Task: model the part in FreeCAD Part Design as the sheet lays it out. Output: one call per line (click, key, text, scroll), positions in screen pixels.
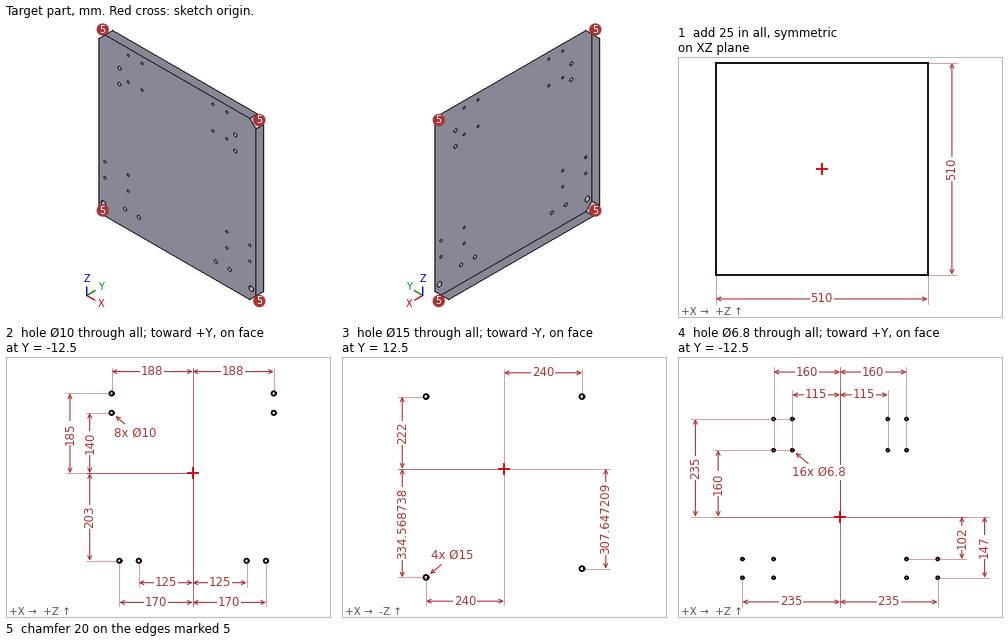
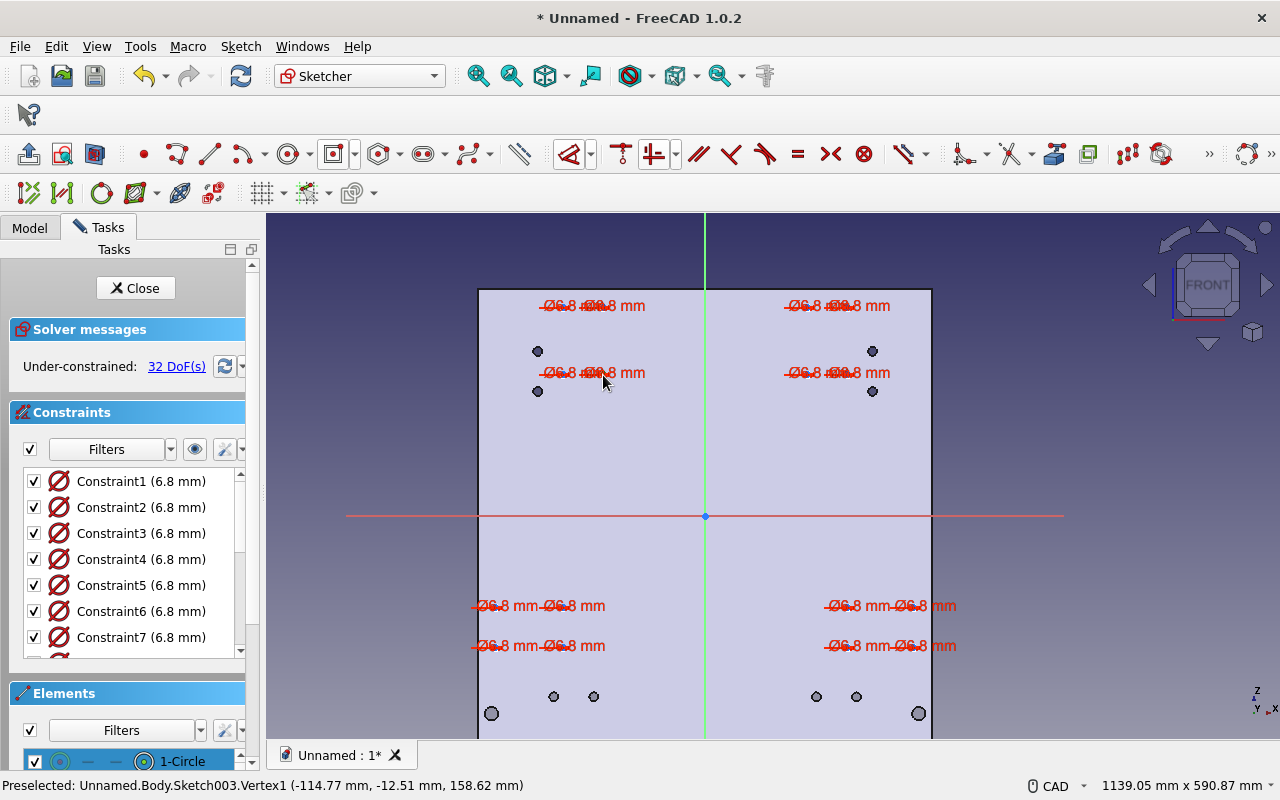
click(563, 375)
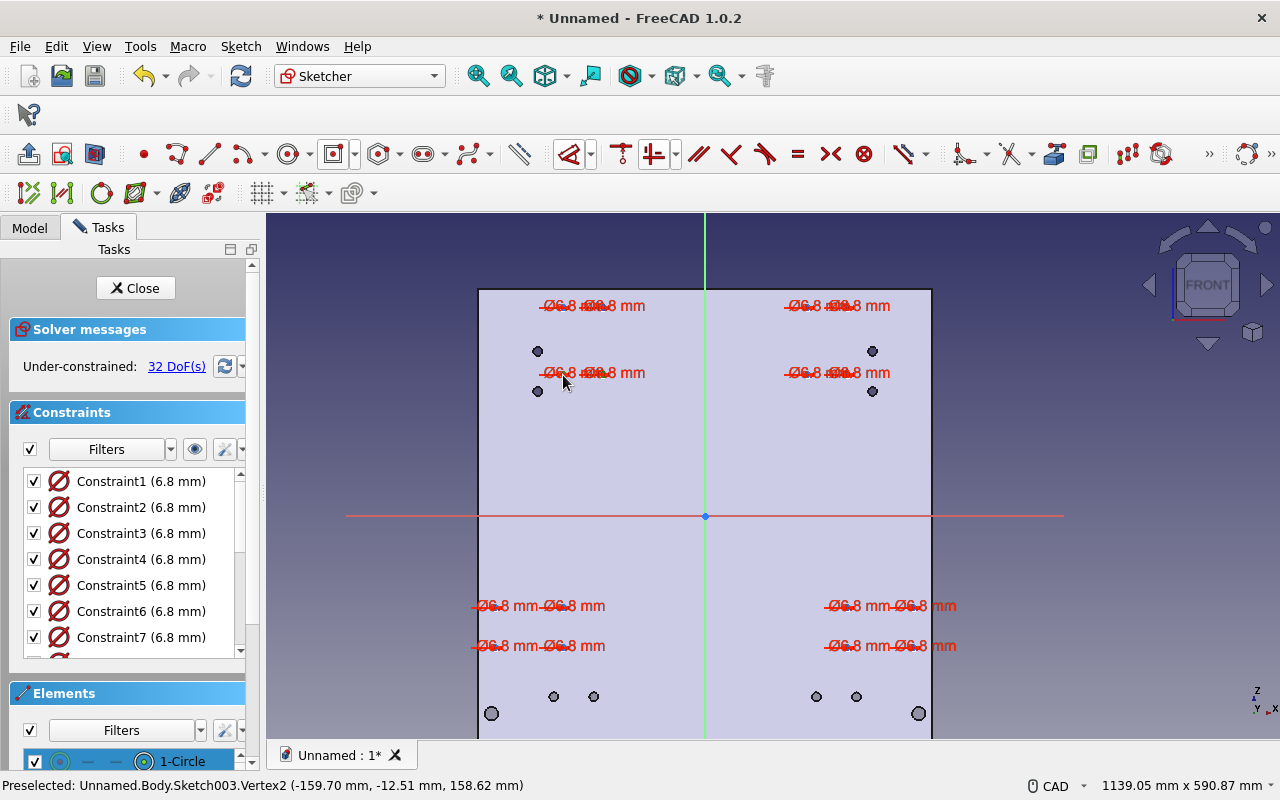
click(676, 154)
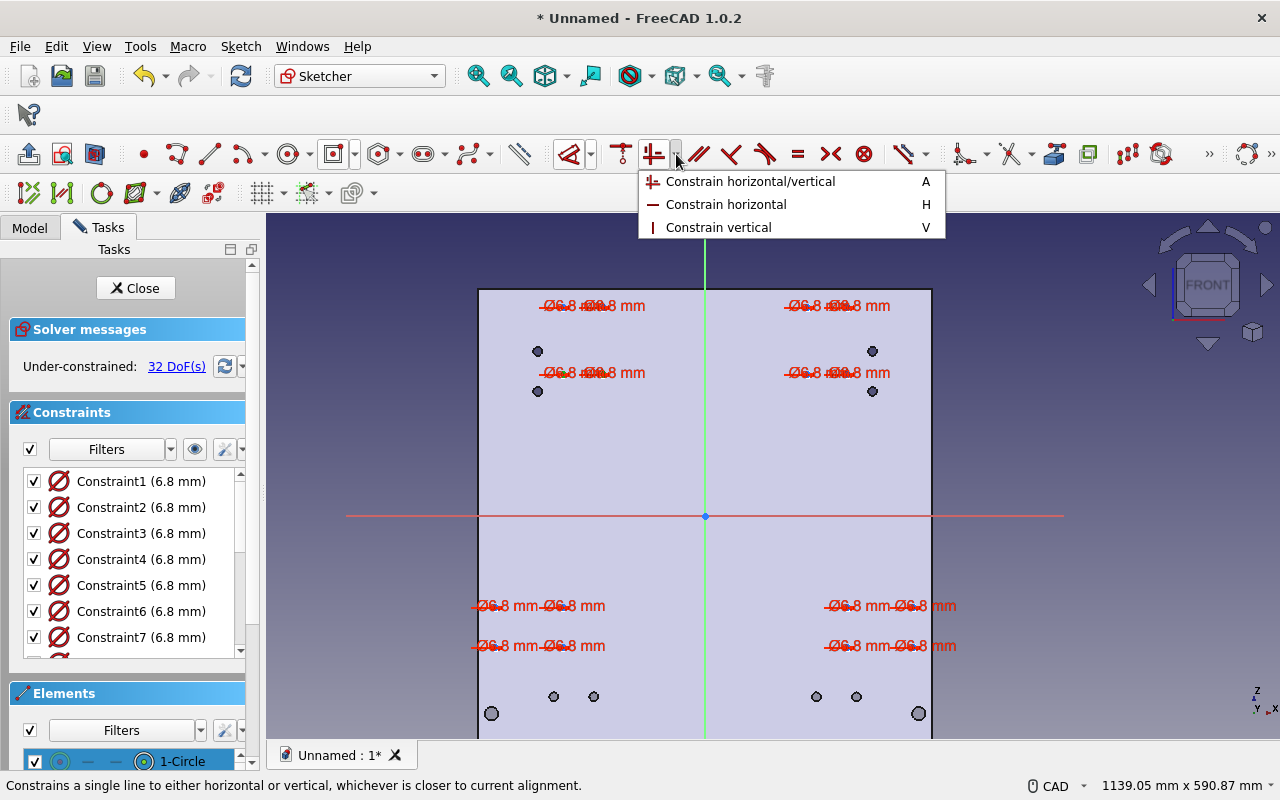
click(792, 204)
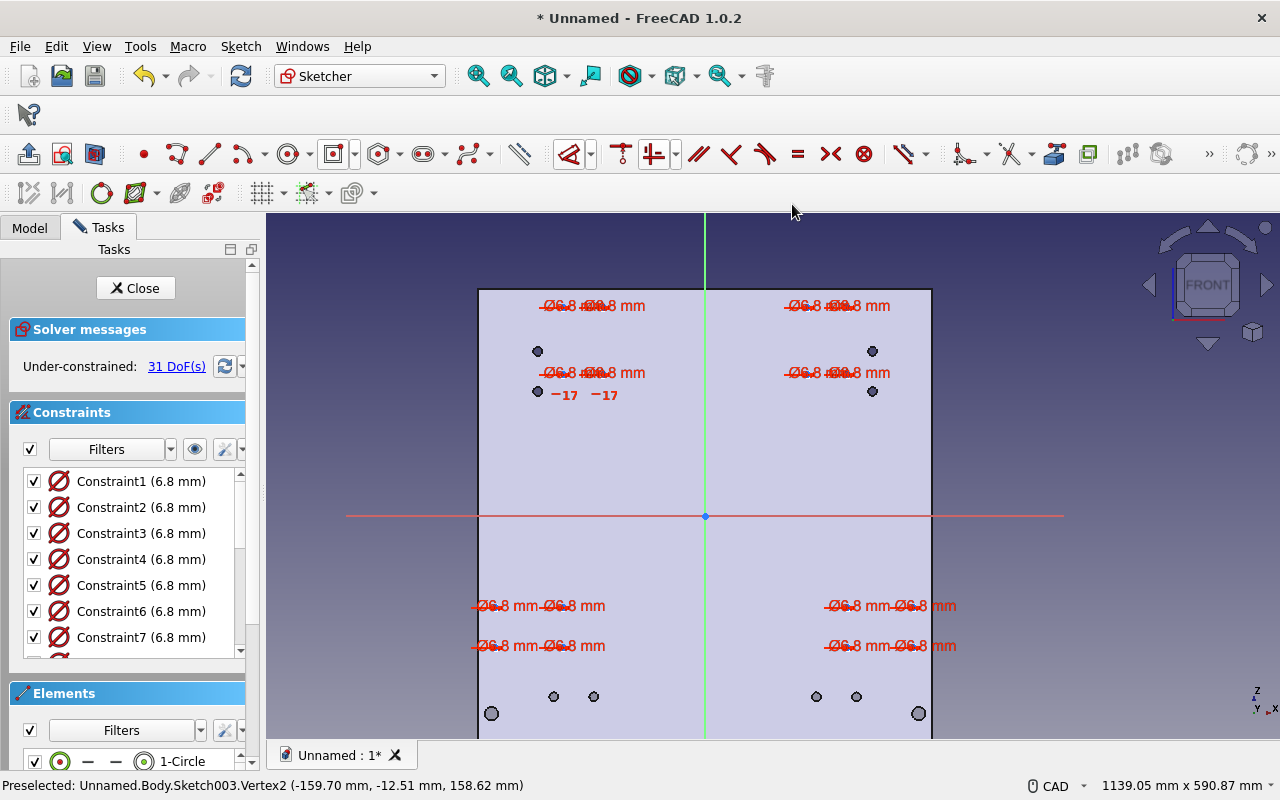
click(603, 375)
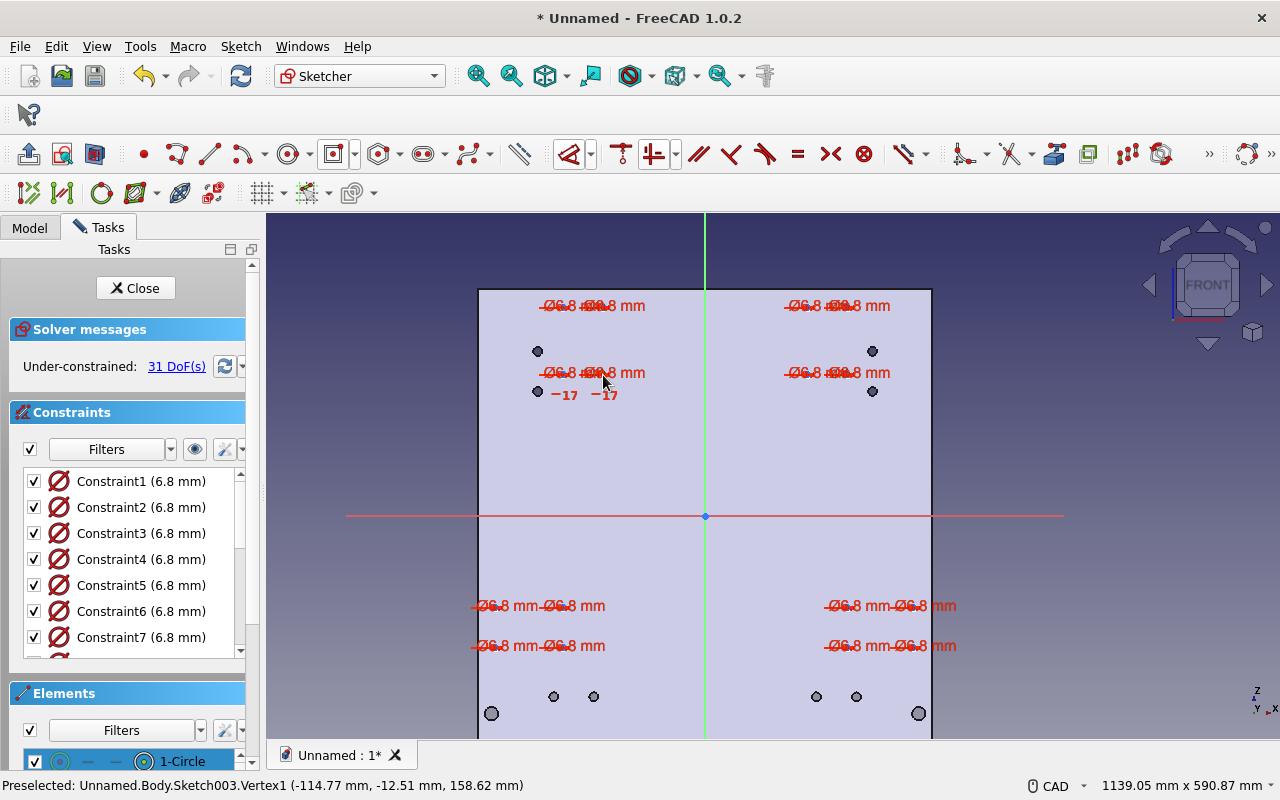
click(603, 308)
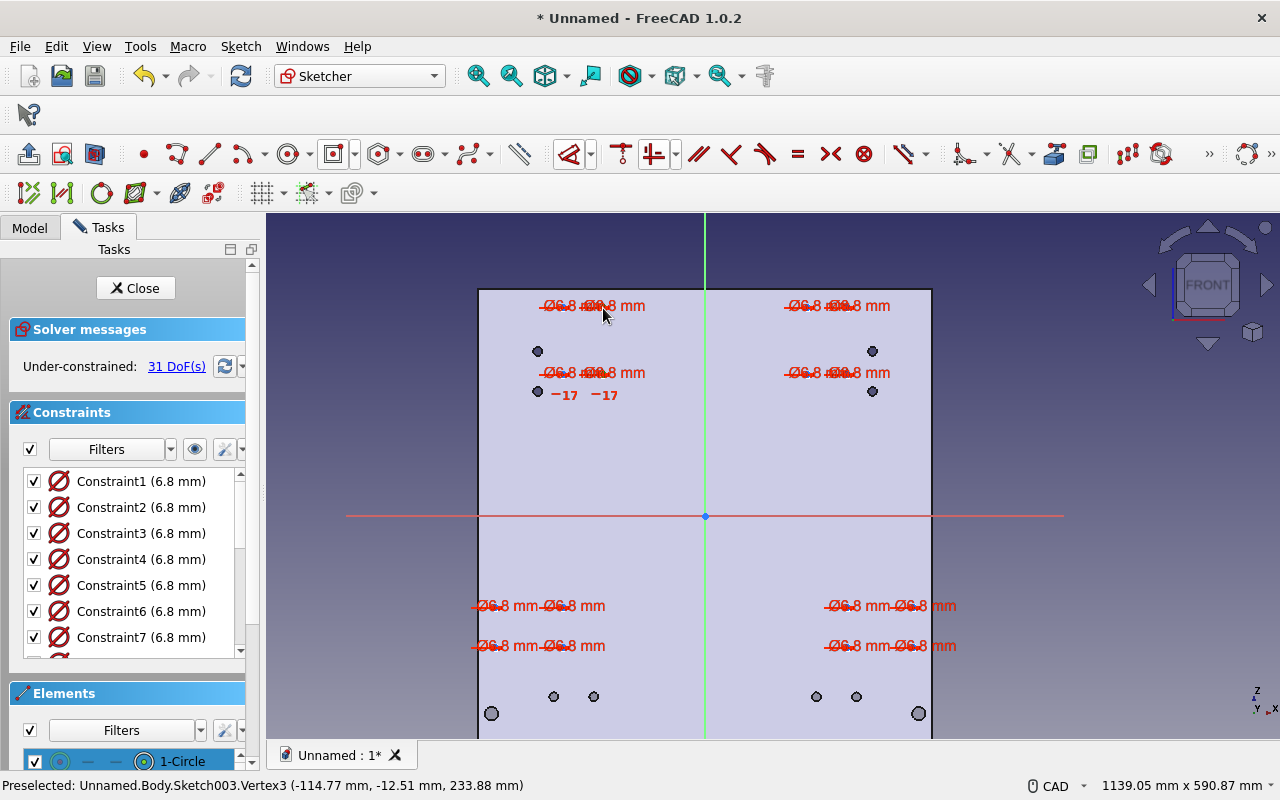
key(v)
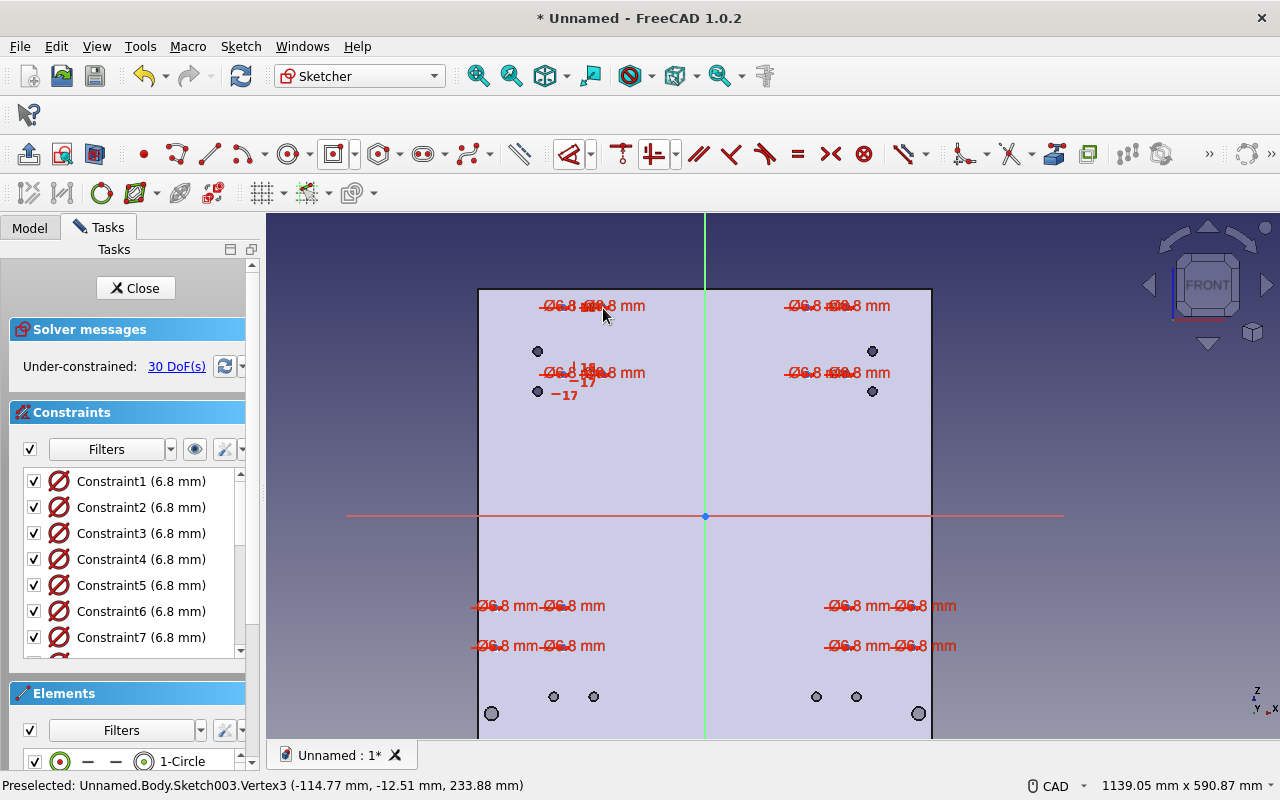
click(563, 375)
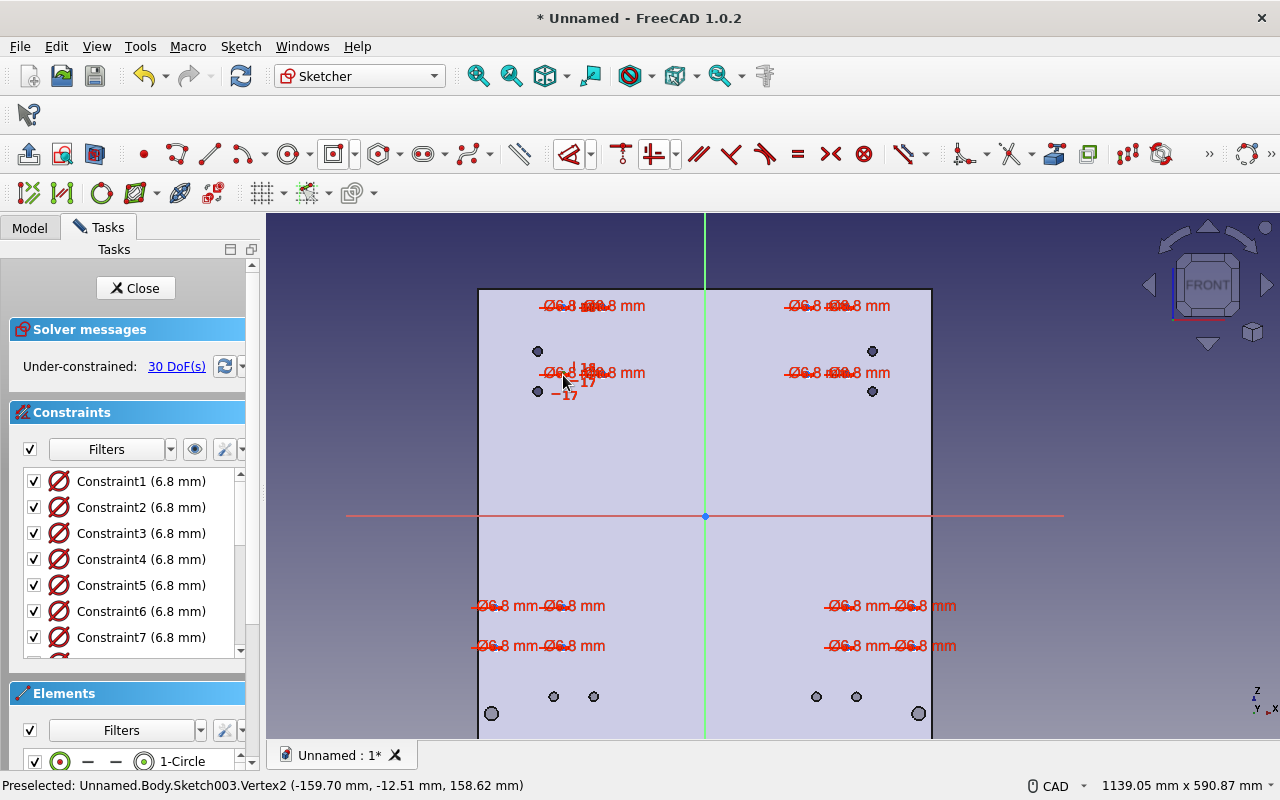
click(563, 308)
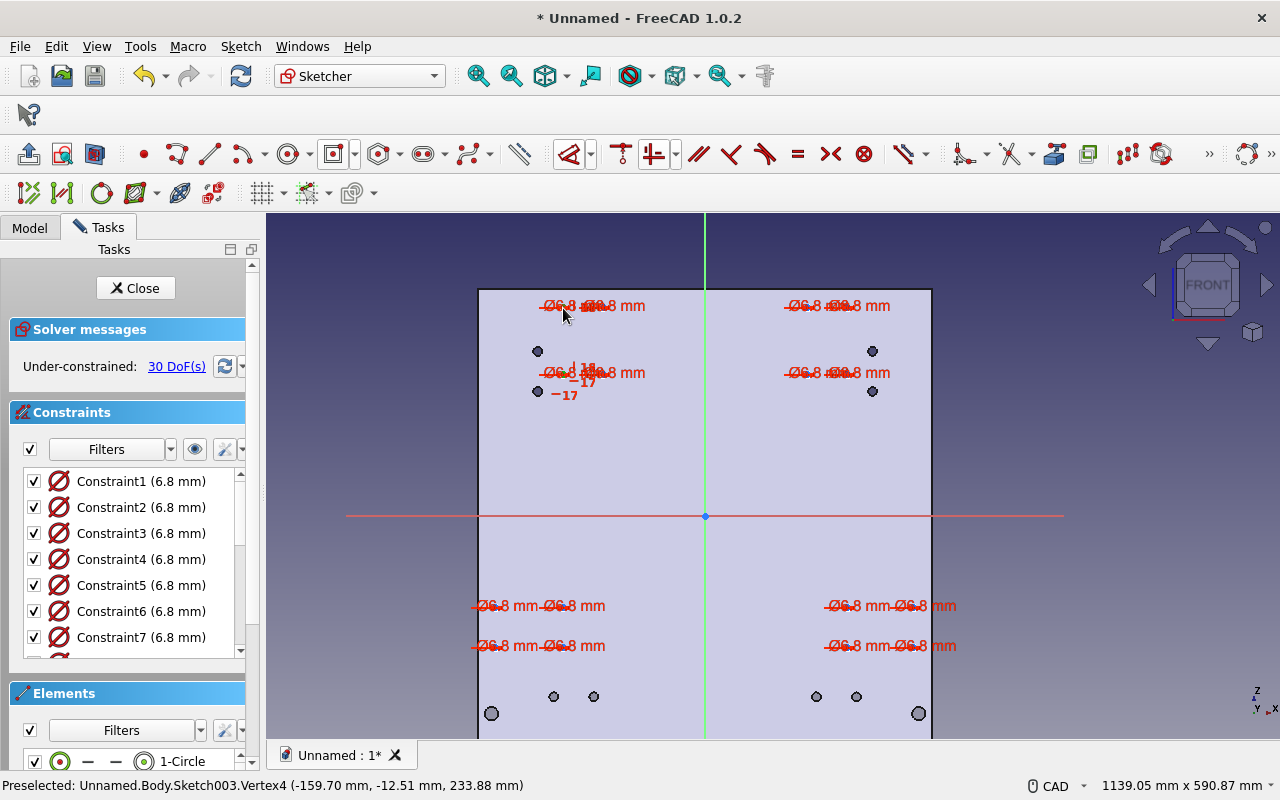
click(676, 154)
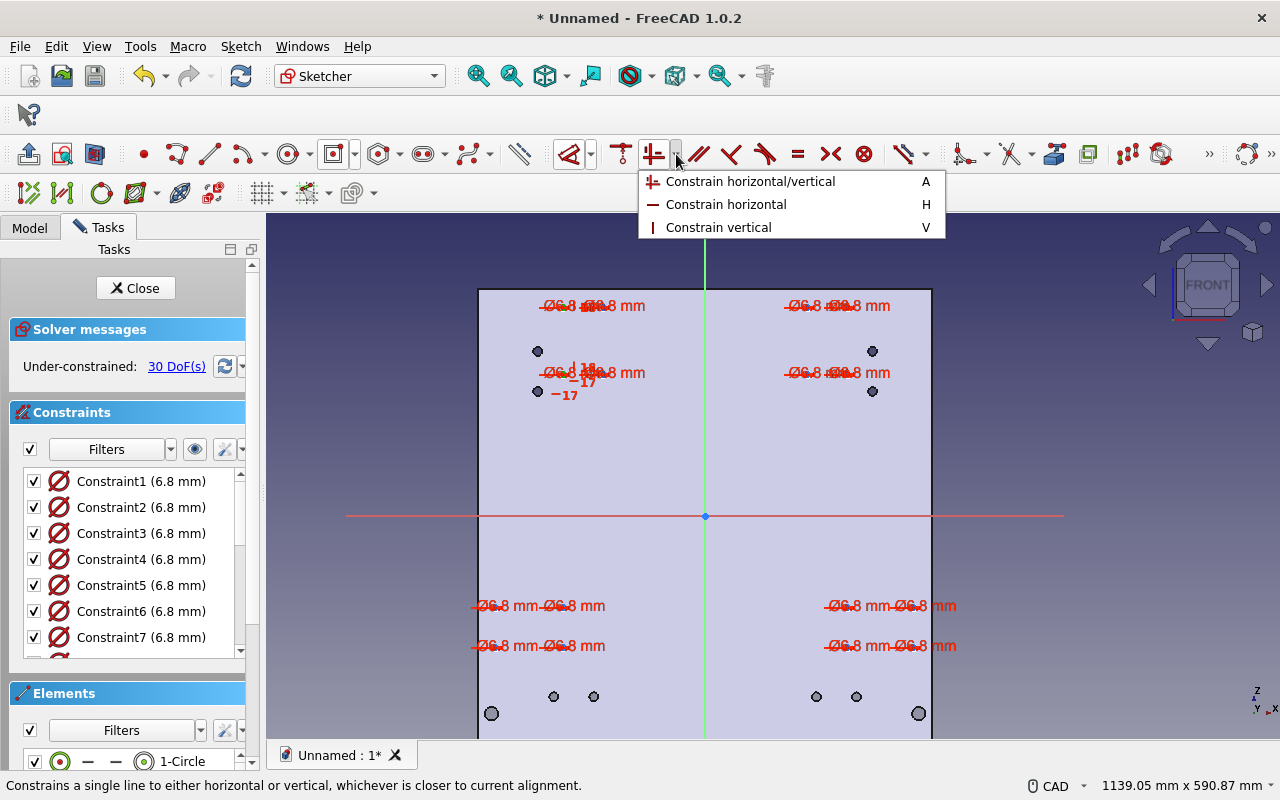
click(792, 228)